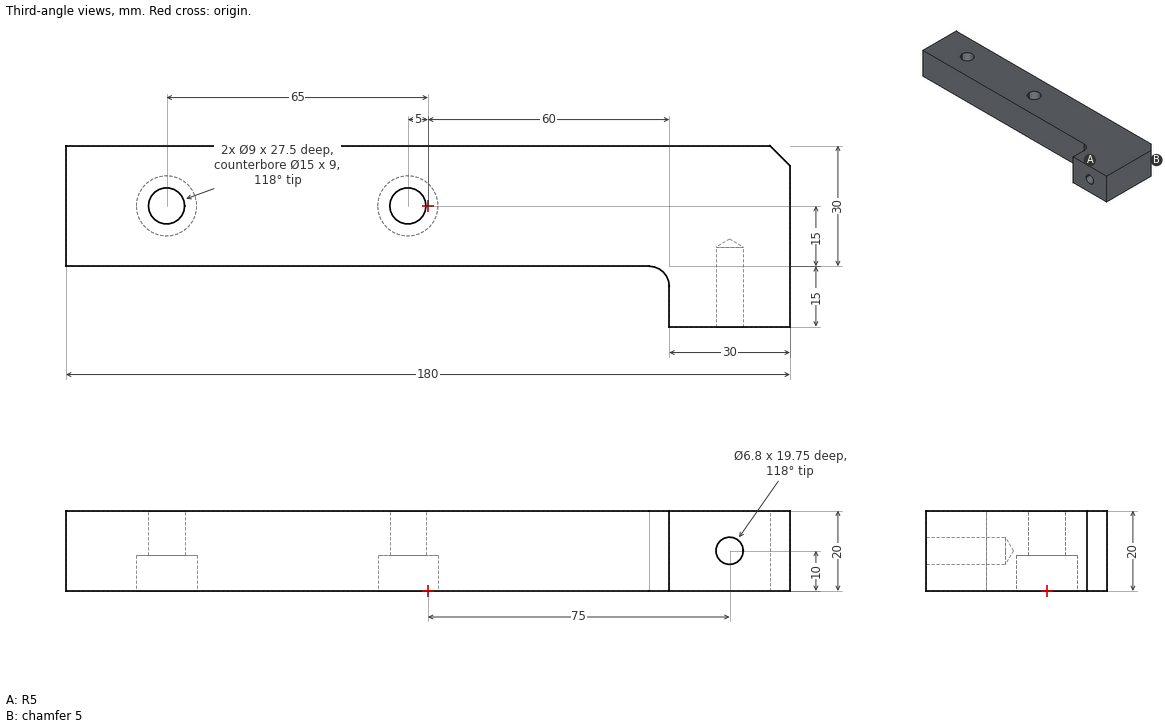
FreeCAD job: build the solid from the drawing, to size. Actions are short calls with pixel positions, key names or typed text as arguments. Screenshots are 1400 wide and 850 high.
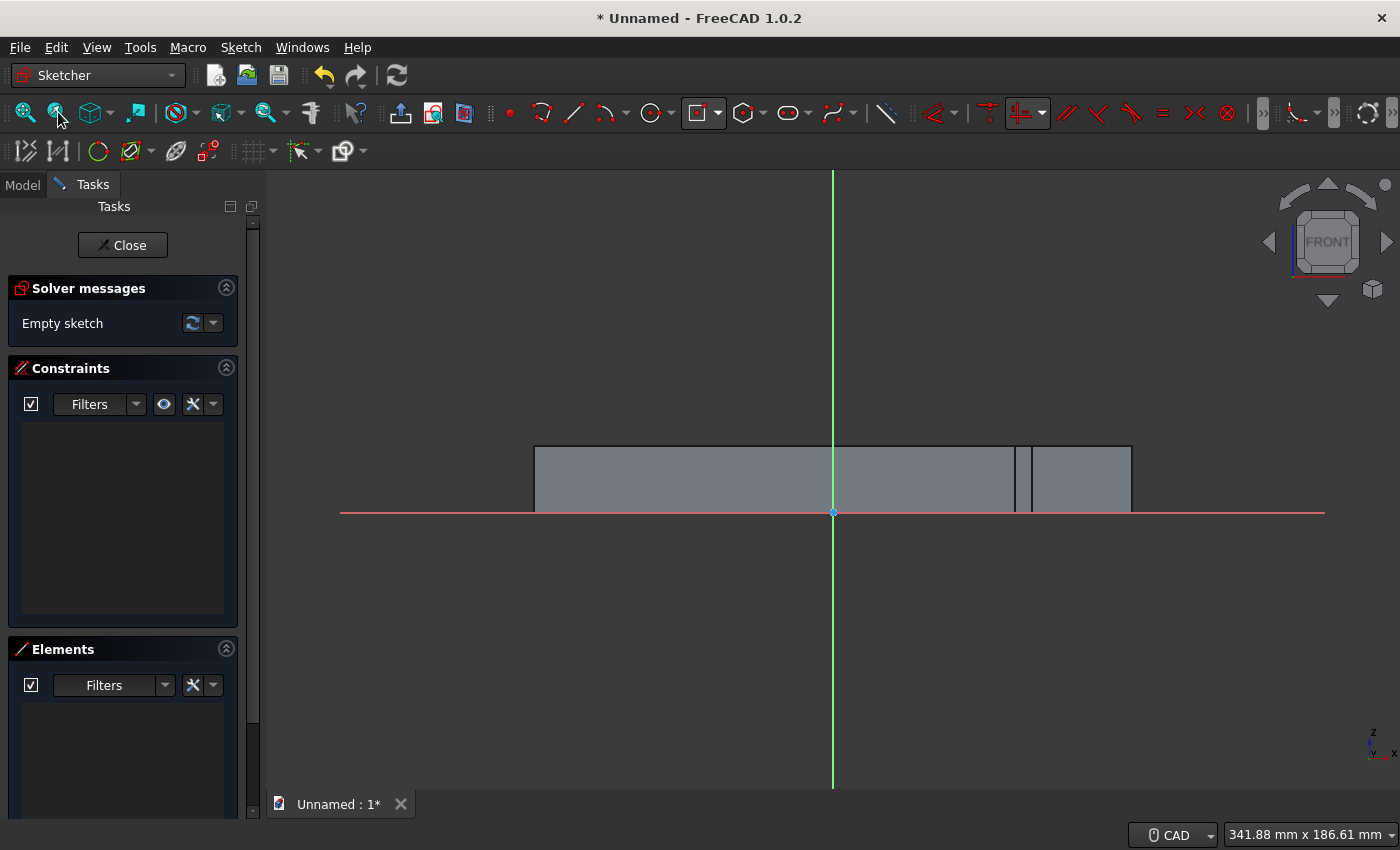
scroll(1102, 479, up, 14)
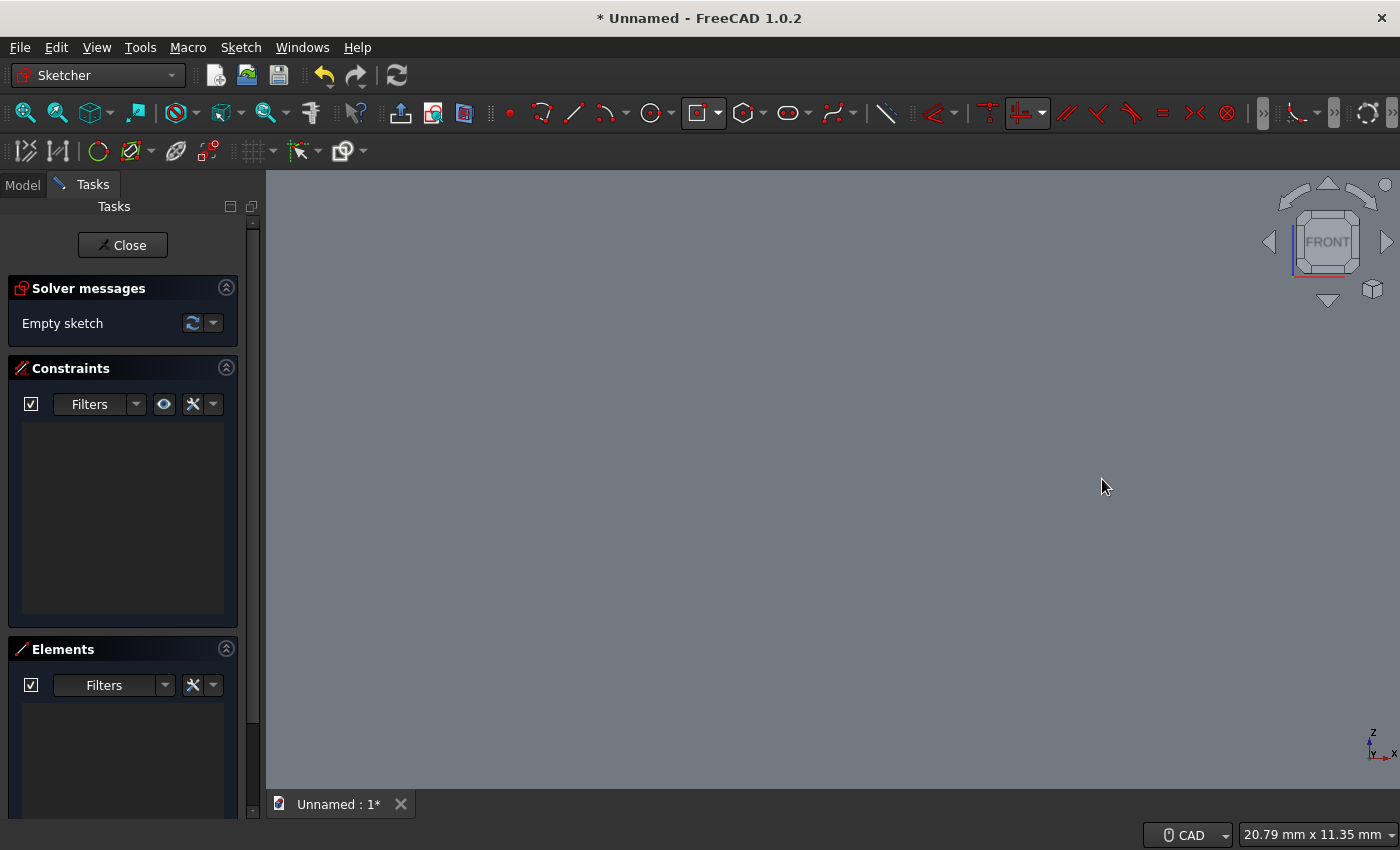
key(g)
key(c)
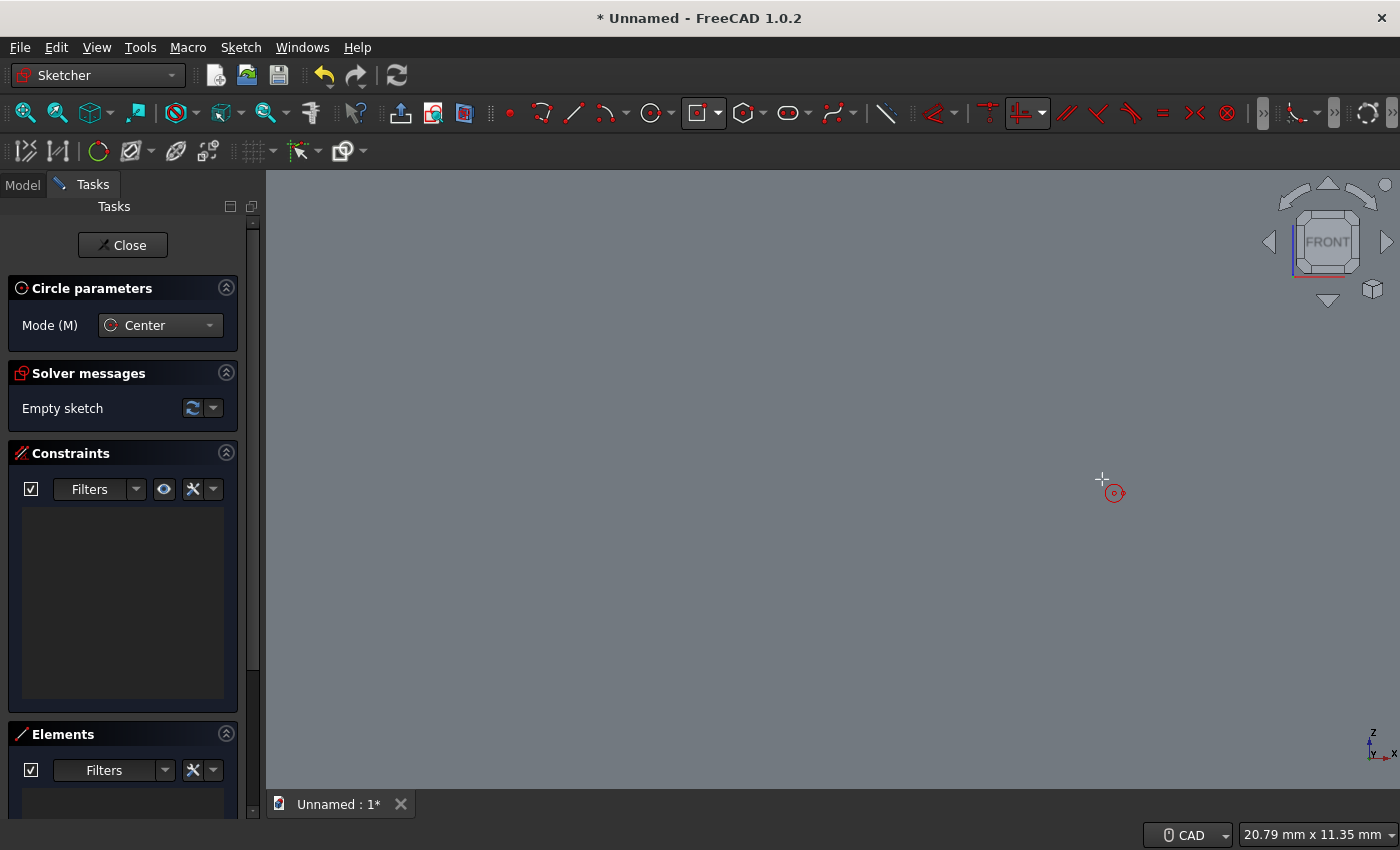
click(758, 479)
move(889, 348)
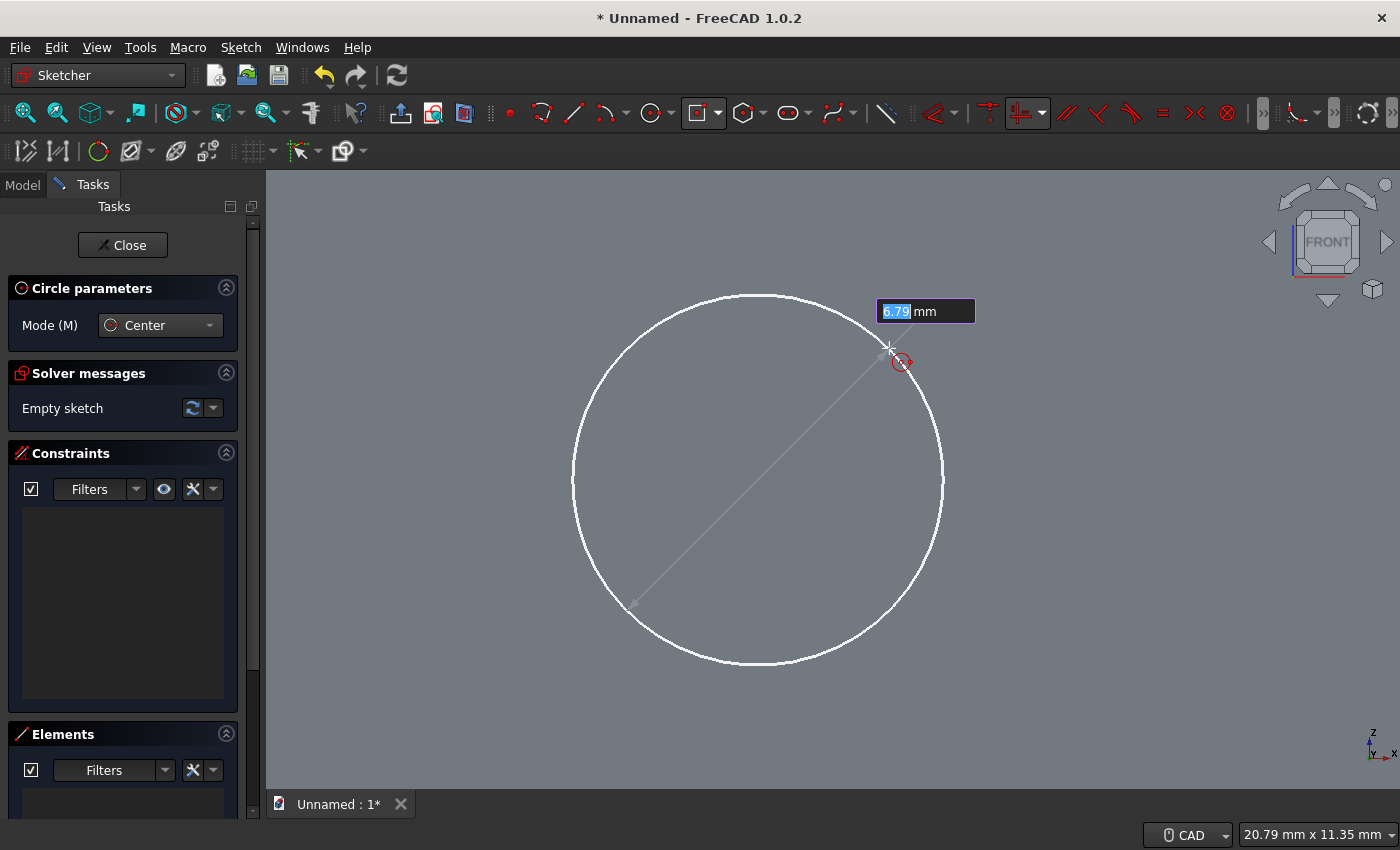
text(6.8)
key(Return)
key(Escape)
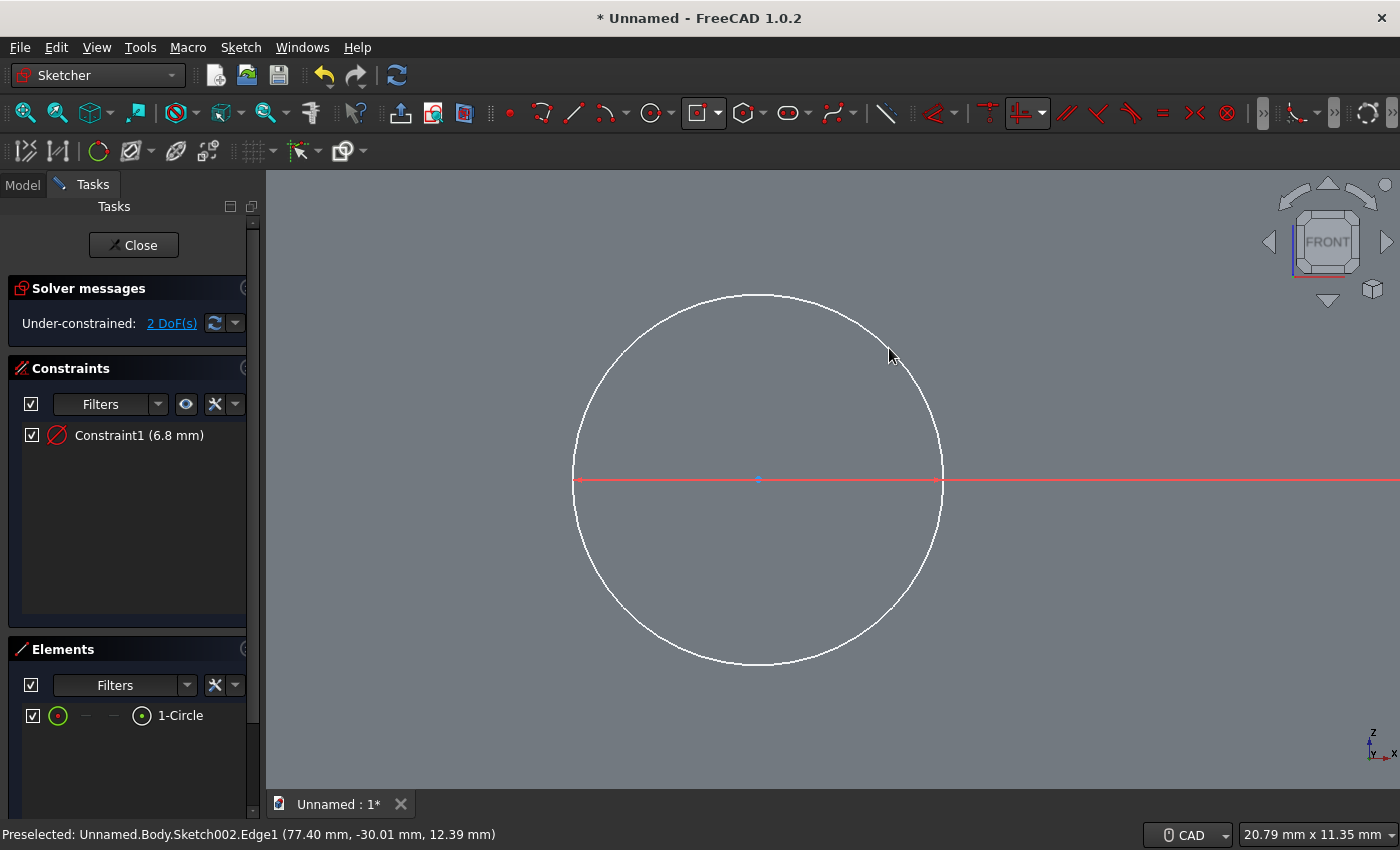
key(d)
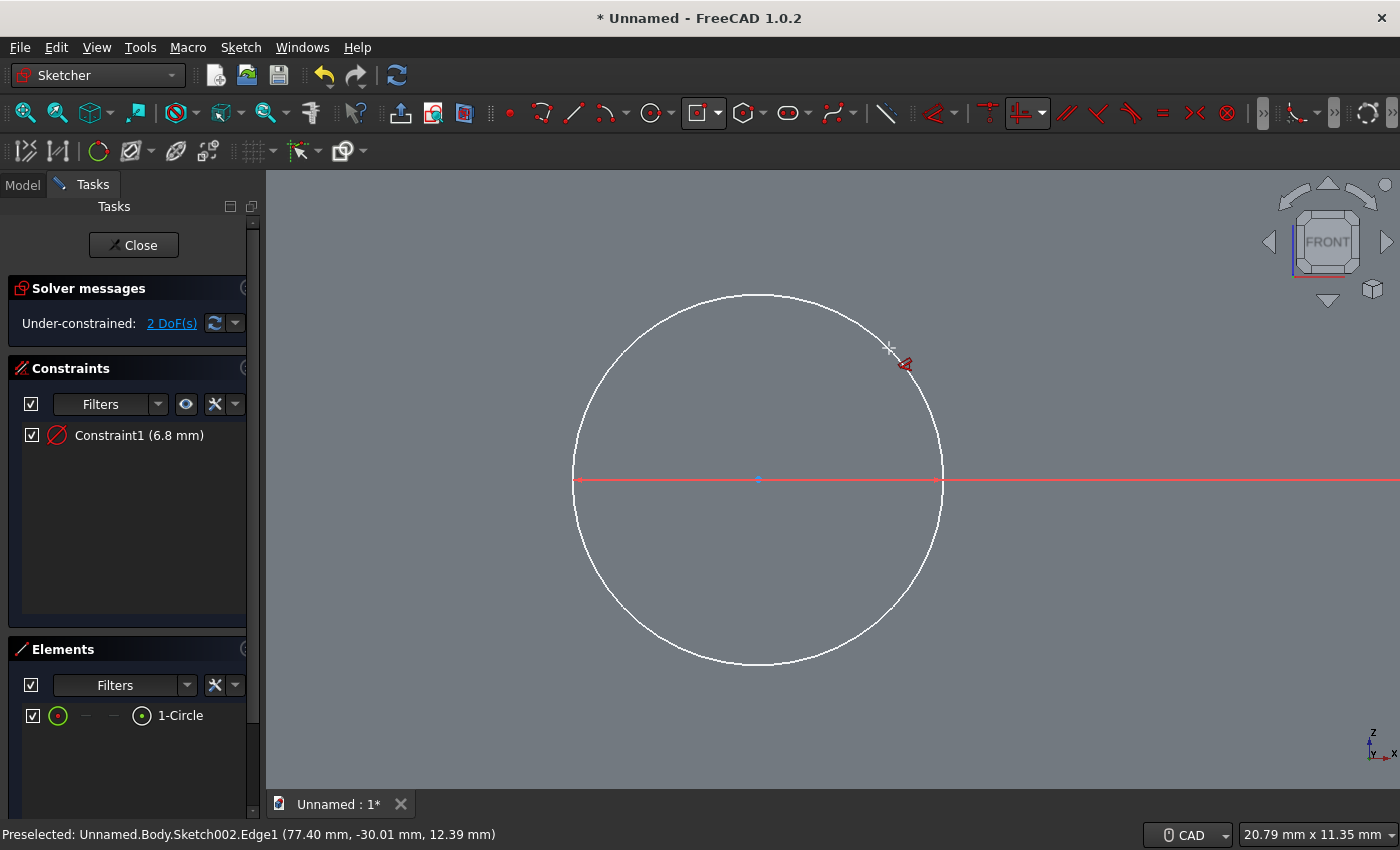
click(758, 480)
click(526, 446)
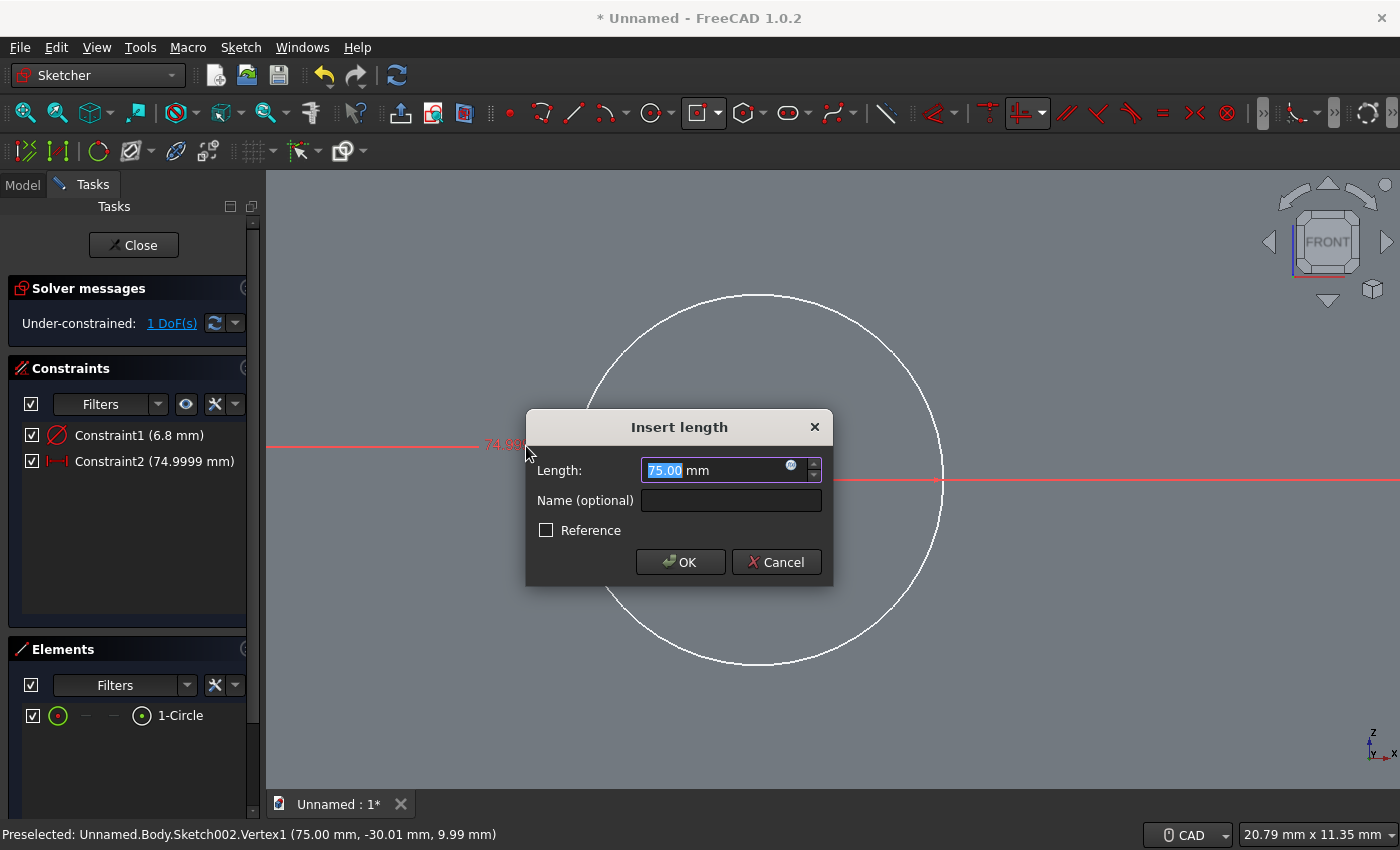
text(75)
key(Return)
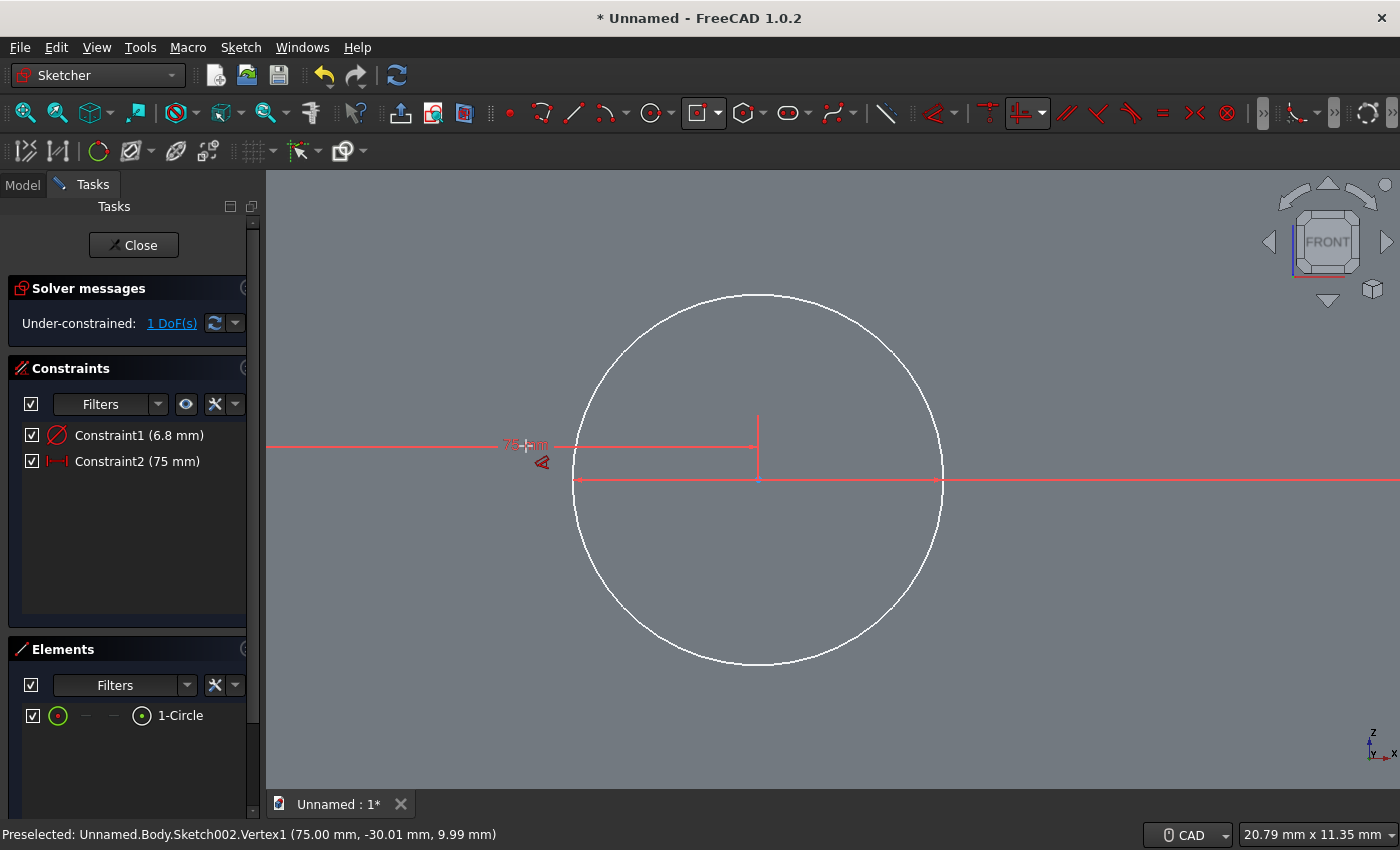
click(758, 480)
click(792, 621)